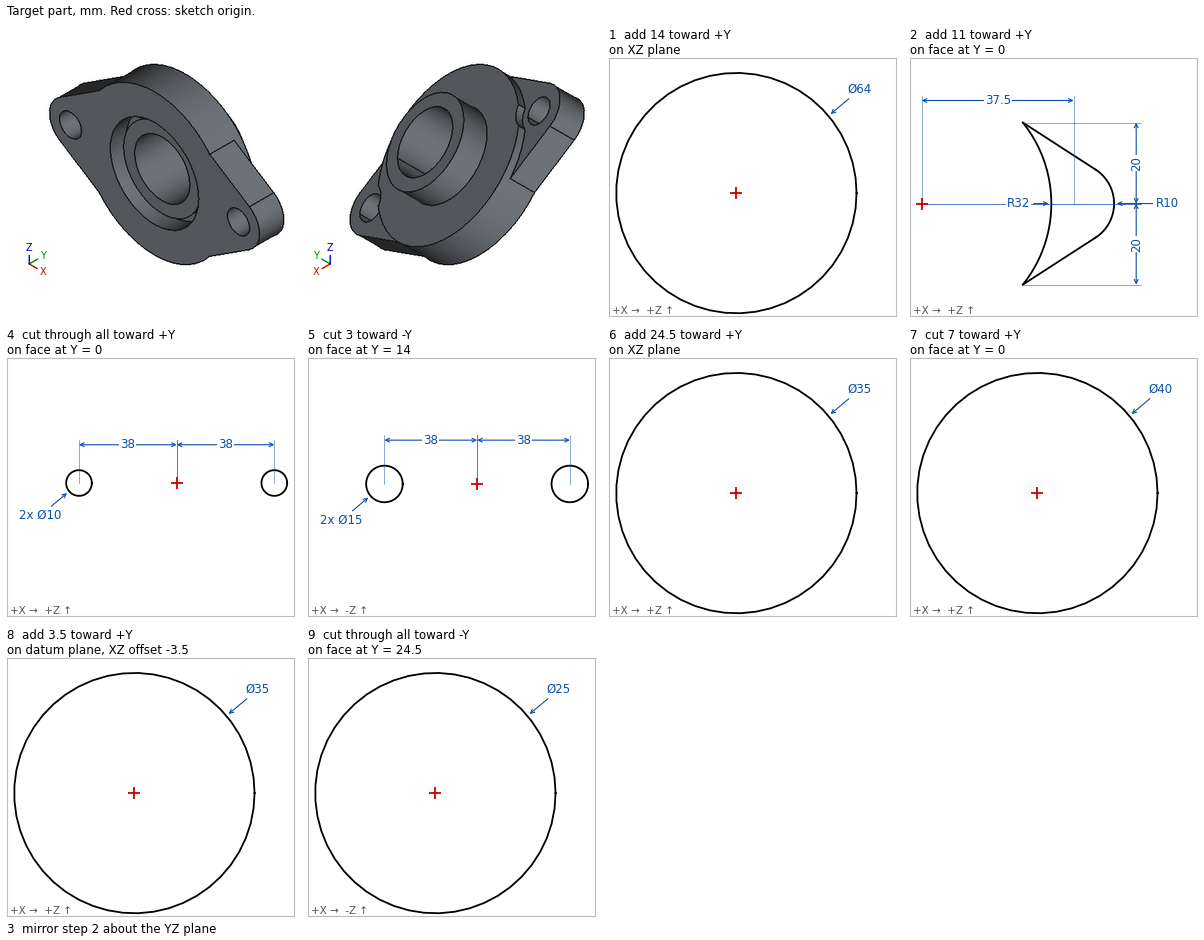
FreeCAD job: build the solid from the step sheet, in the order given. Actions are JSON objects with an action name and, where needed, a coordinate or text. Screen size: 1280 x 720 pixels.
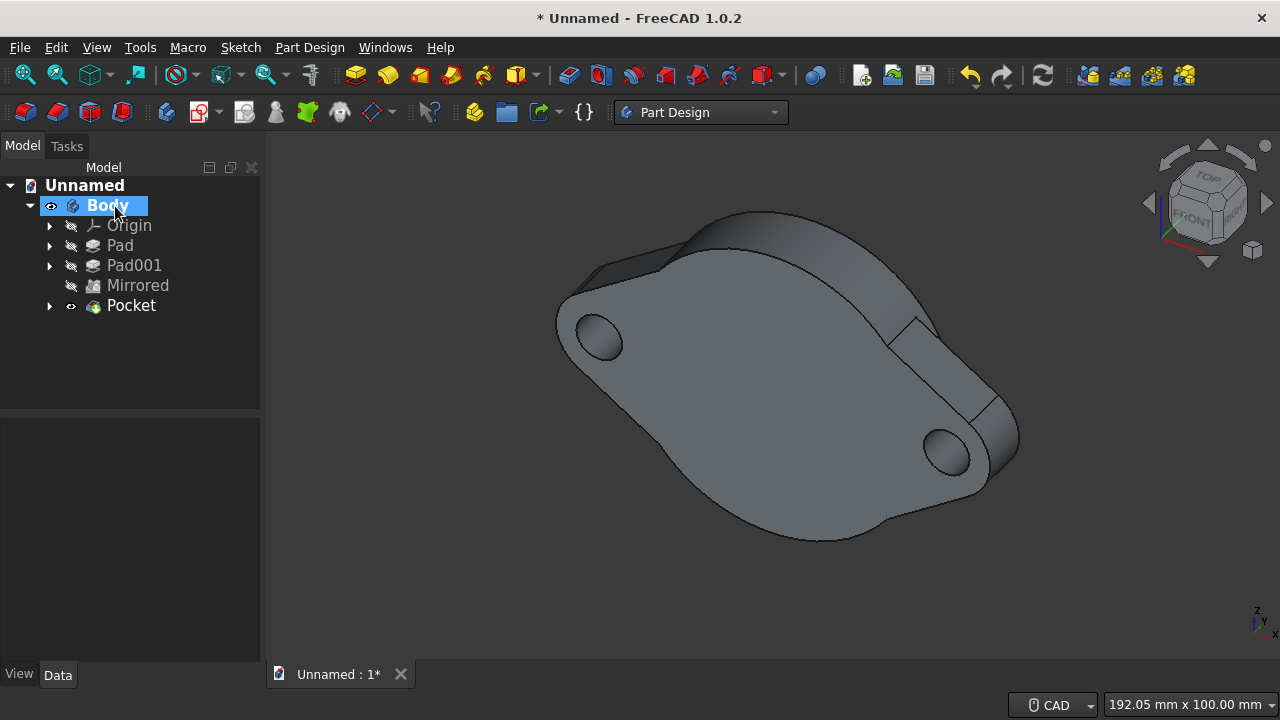
{"action": "key", "text": "4"}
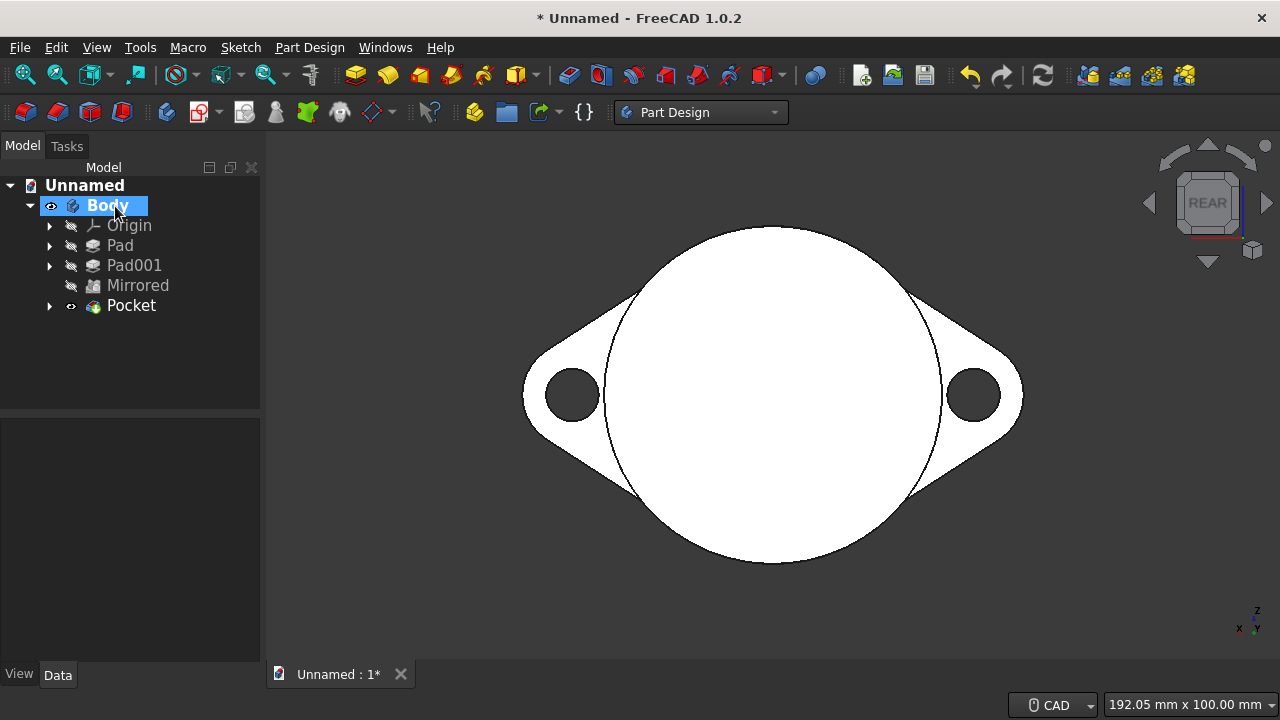
{"action": "left_click", "coordinate": [773, 394]}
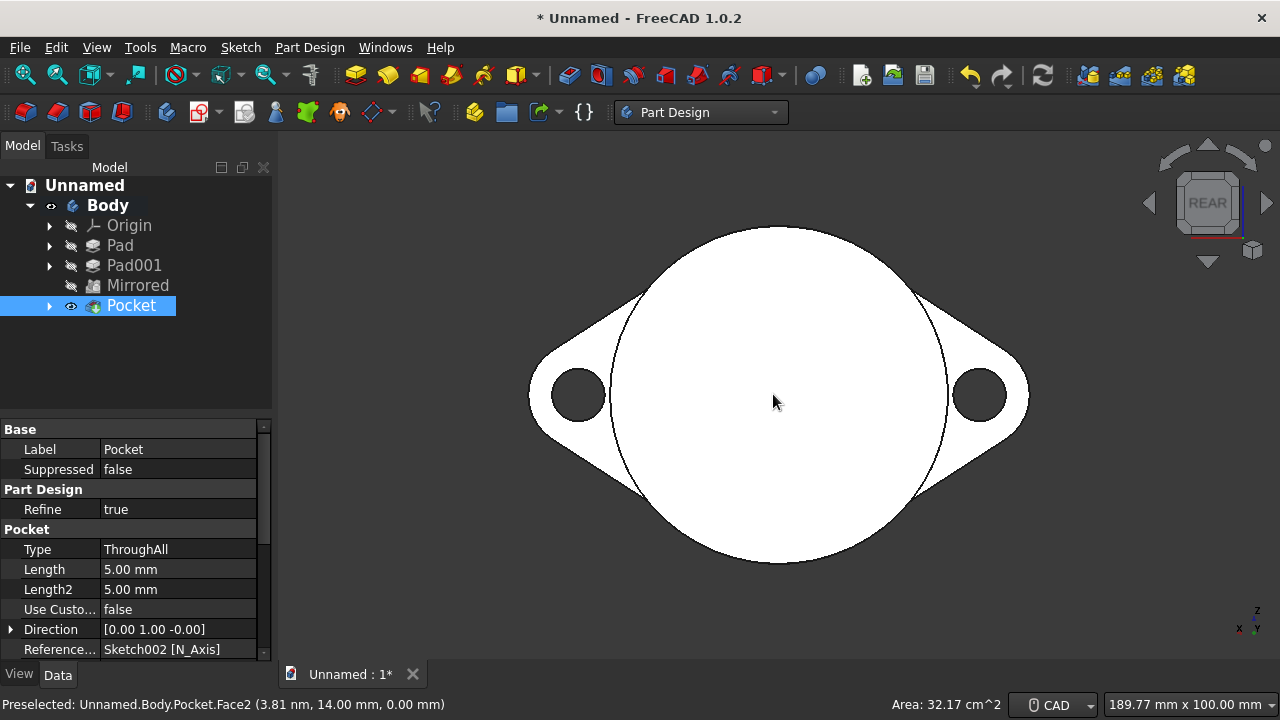
{"action": "left_click", "coordinate": [200, 112]}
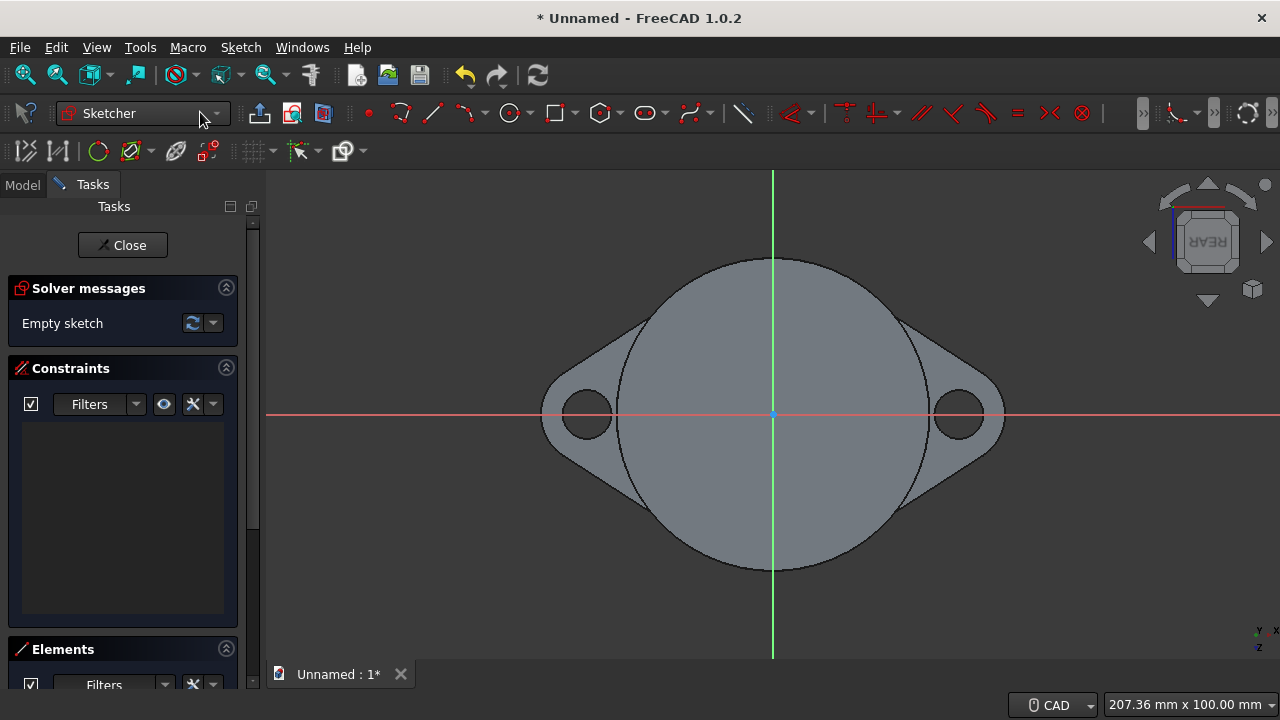
{"action": "key", "text": "g c"}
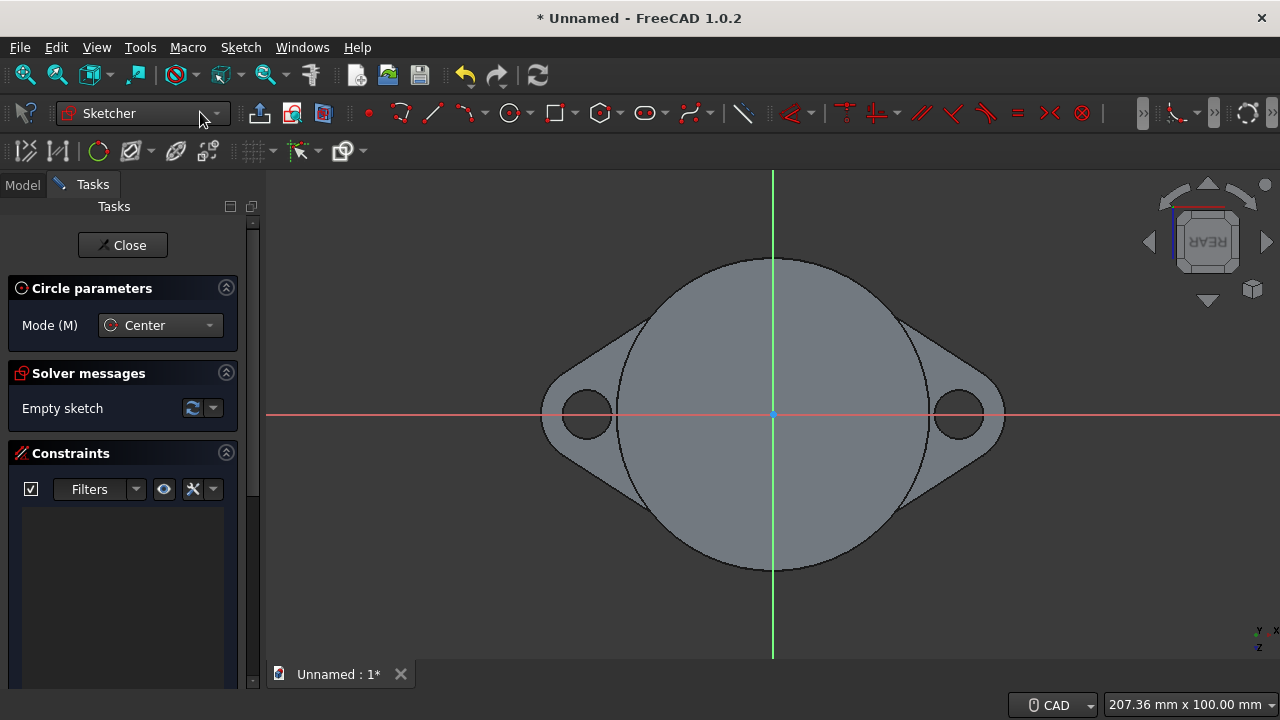
{"action": "left_click", "coordinate": [587, 415]}
{"action": "left_click", "coordinate": [613, 389]}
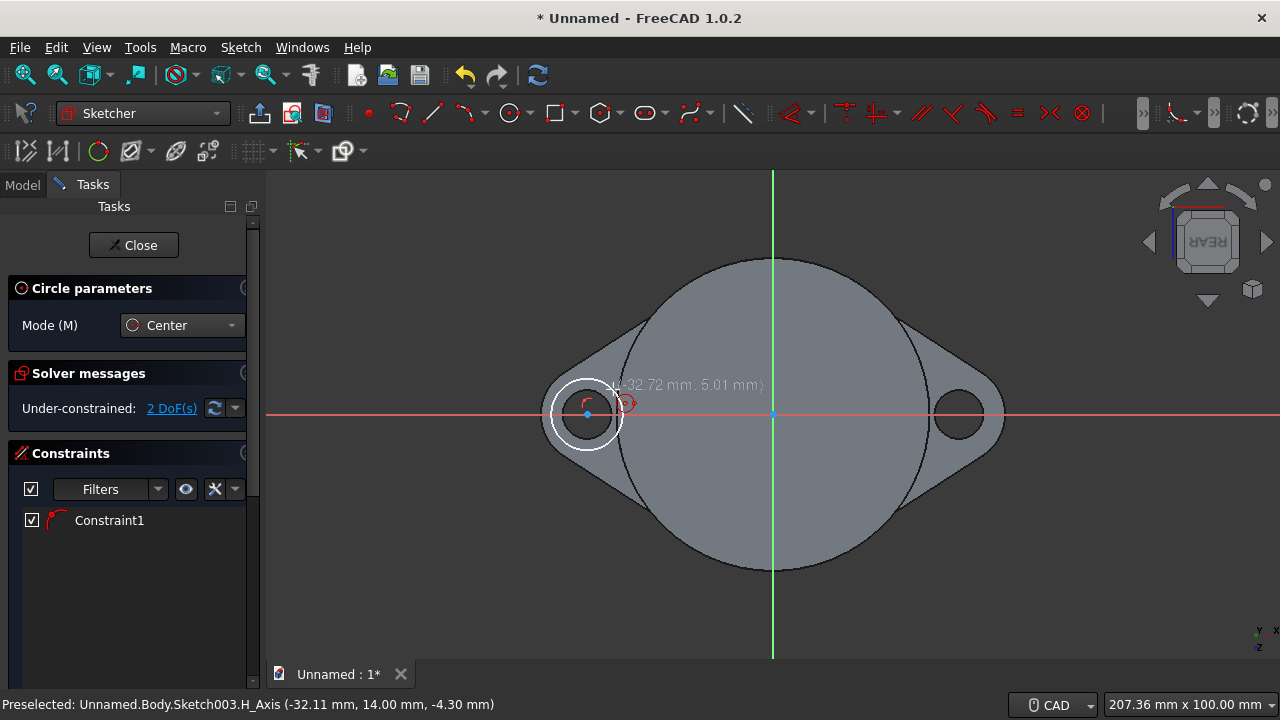
{"action": "left_click", "coordinate": [959, 415]}
{"action": "left_click", "coordinate": [985, 389]}
{"action": "key", "text": "Escape"}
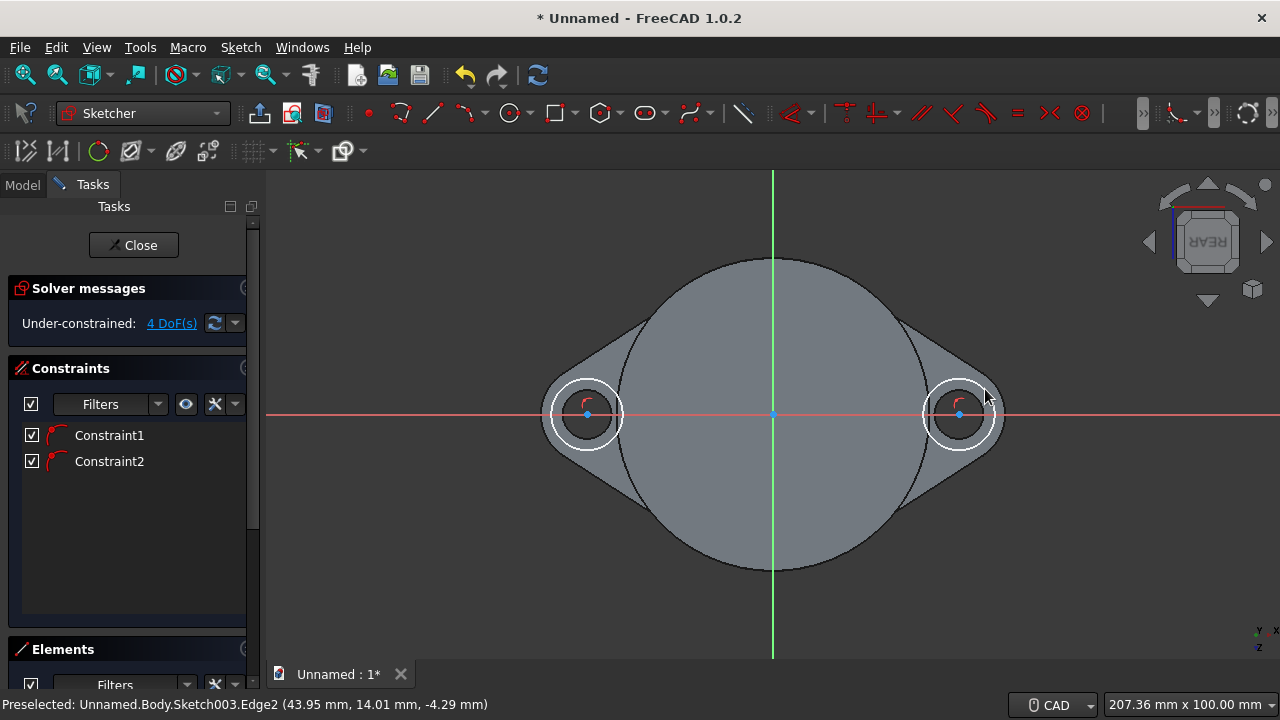
{"action": "left_click", "coordinate": [612, 389]}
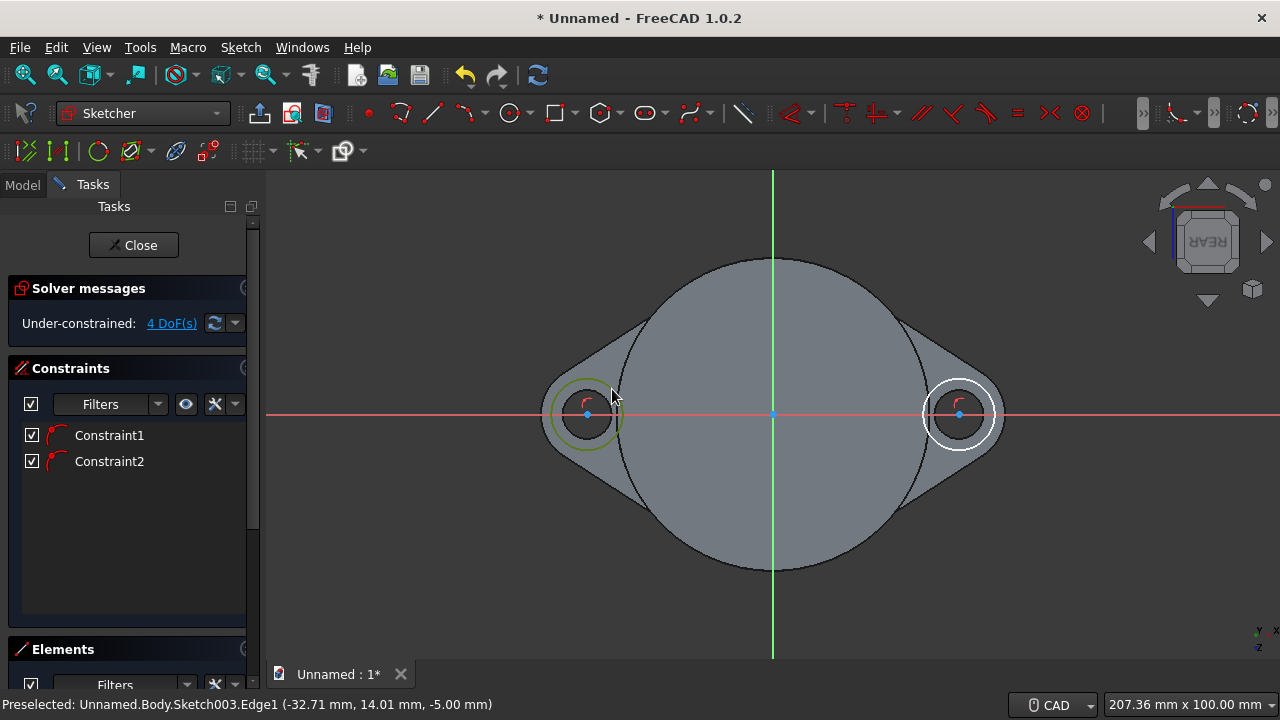
{"action": "left_click", "coordinate": [984, 389]}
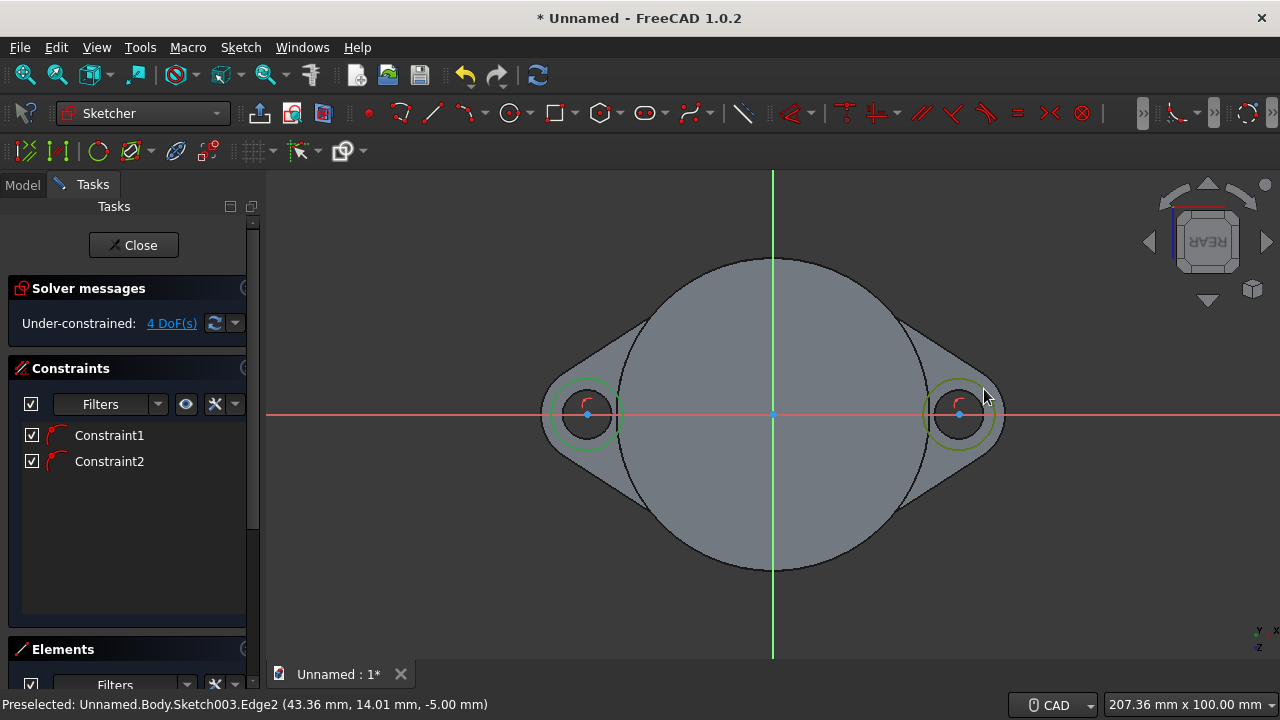
{"action": "left_click", "coordinate": [1018, 114]}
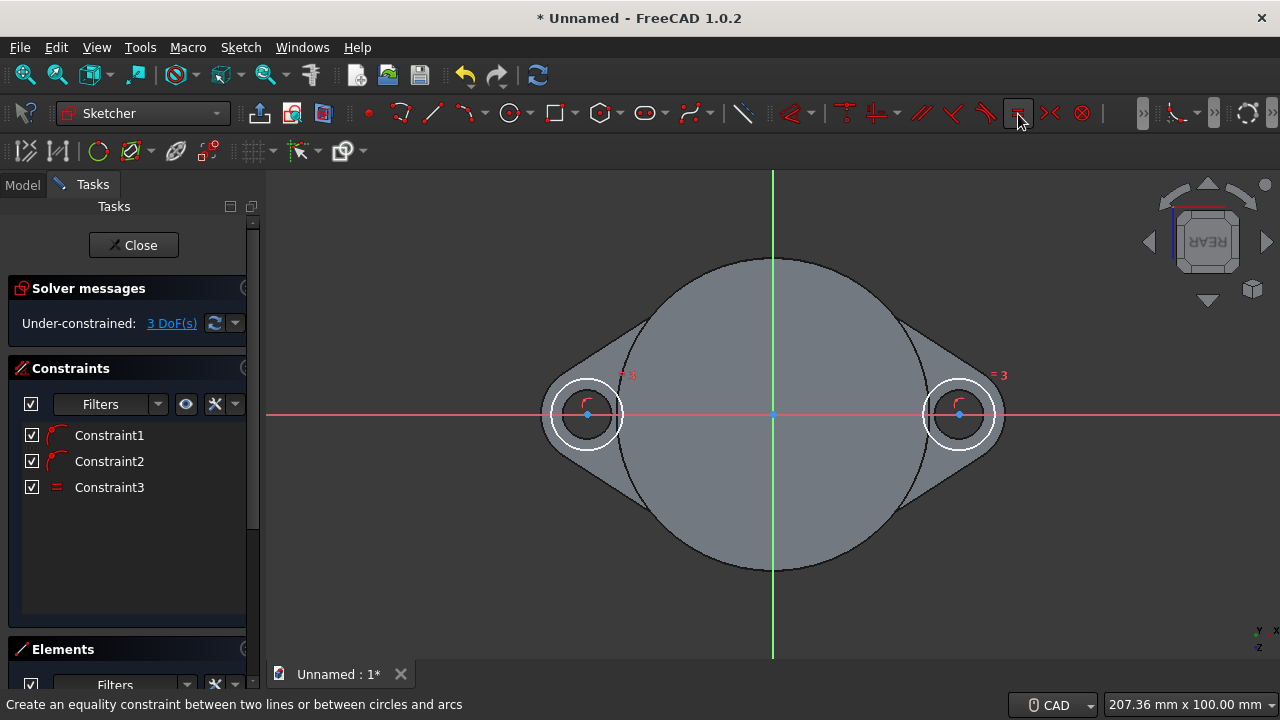
{"action": "key", "text": "d"}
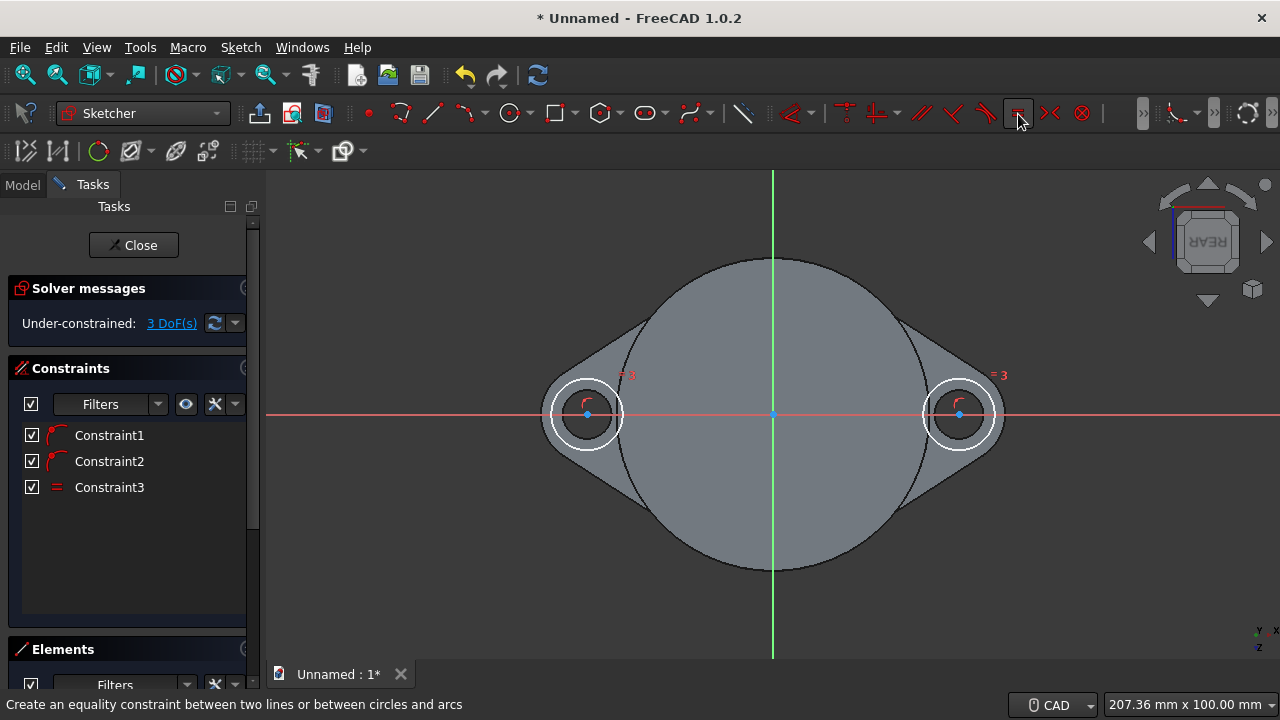
{"action": "left_click", "coordinate": [612, 389]}
{"action": "left_click", "coordinate": [634, 366]}